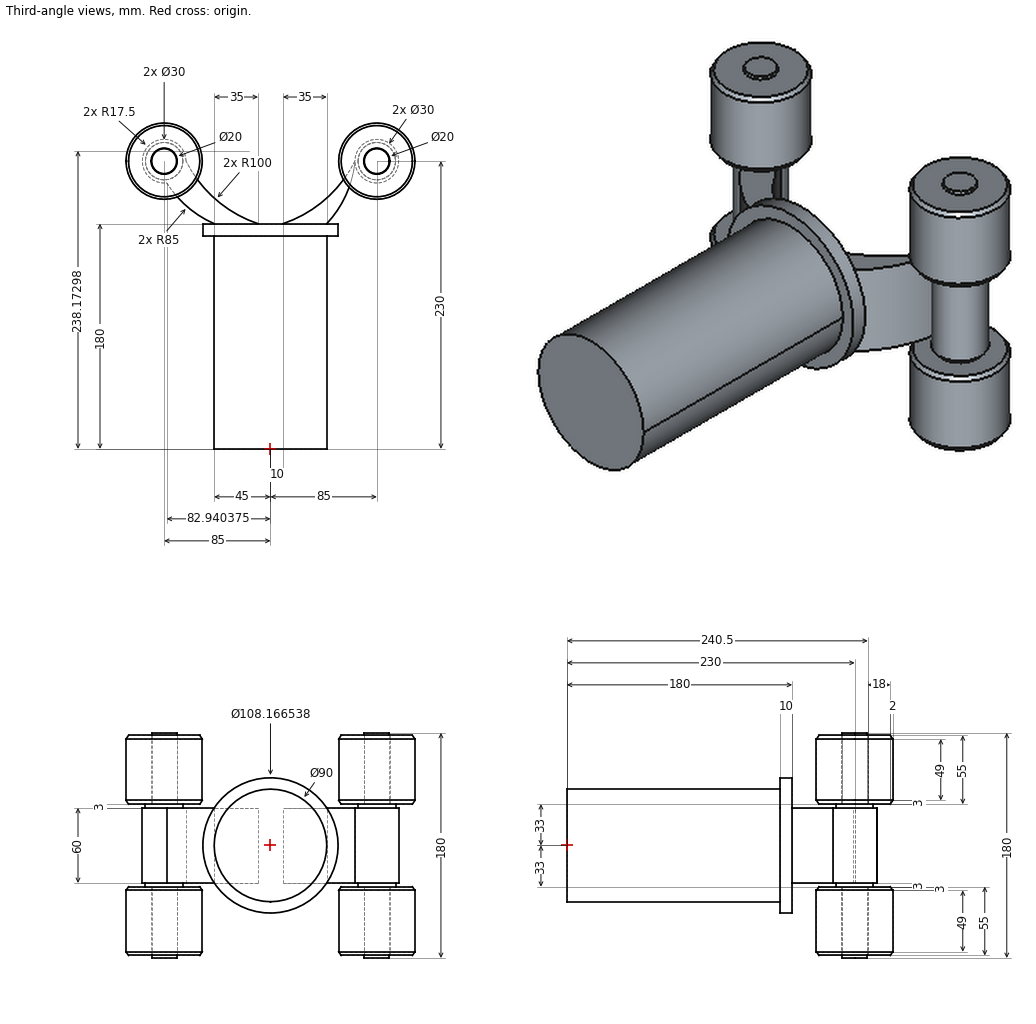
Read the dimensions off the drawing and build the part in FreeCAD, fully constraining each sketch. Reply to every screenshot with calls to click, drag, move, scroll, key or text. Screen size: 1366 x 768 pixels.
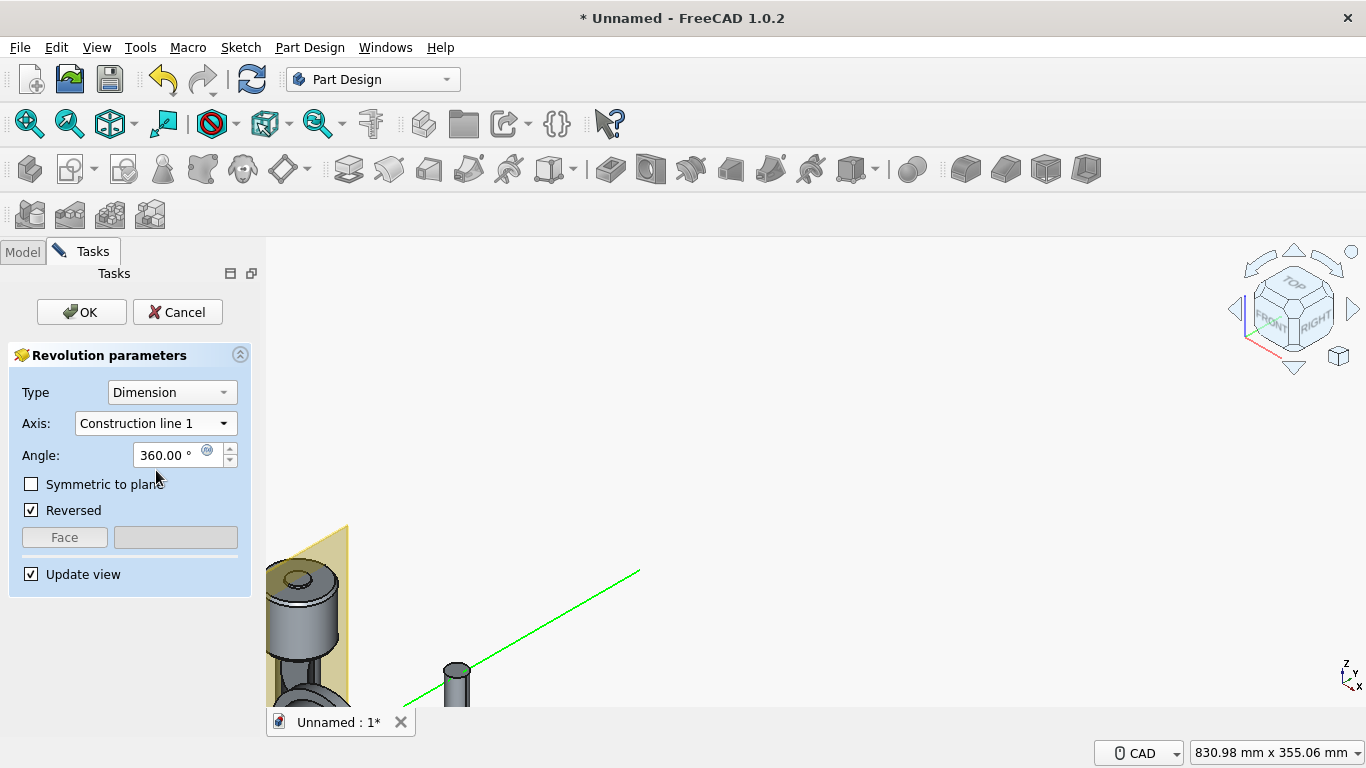
click(82, 312)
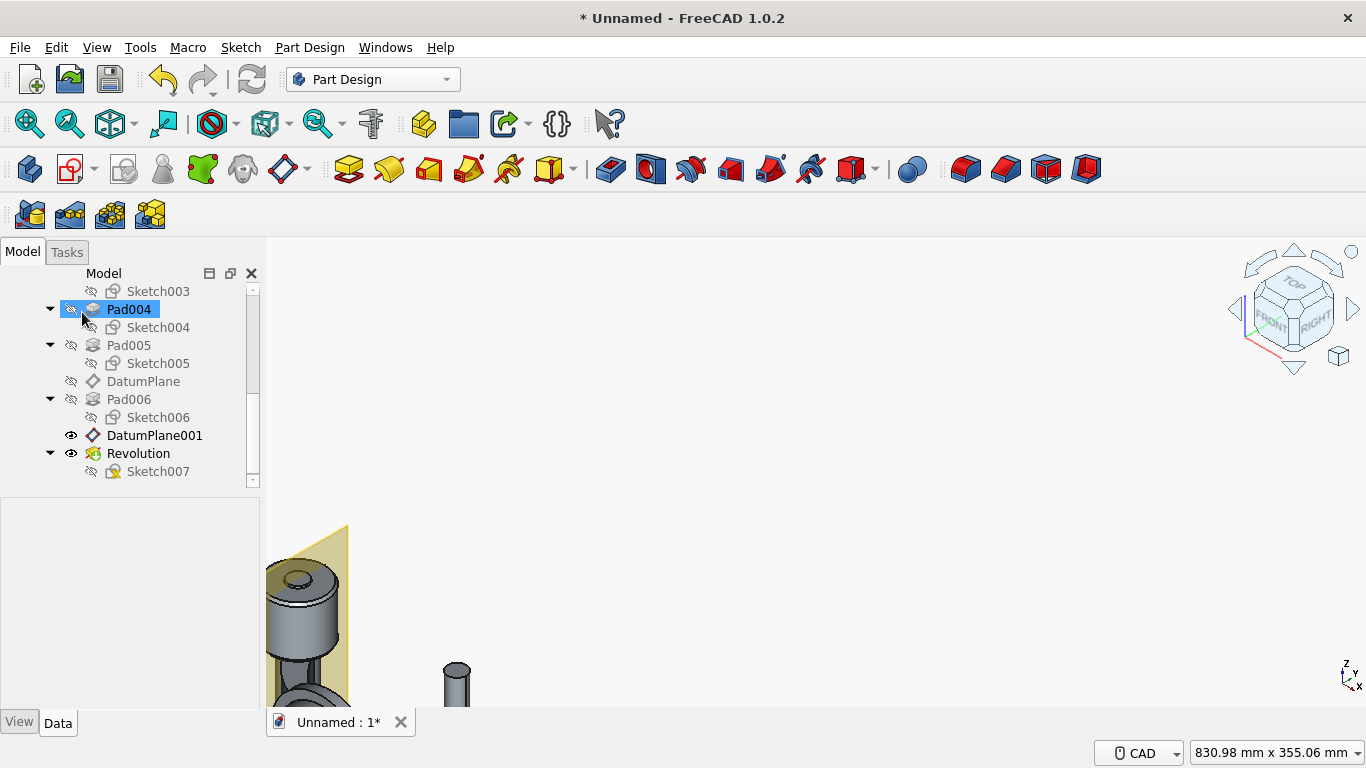
click(116, 435)
key(space)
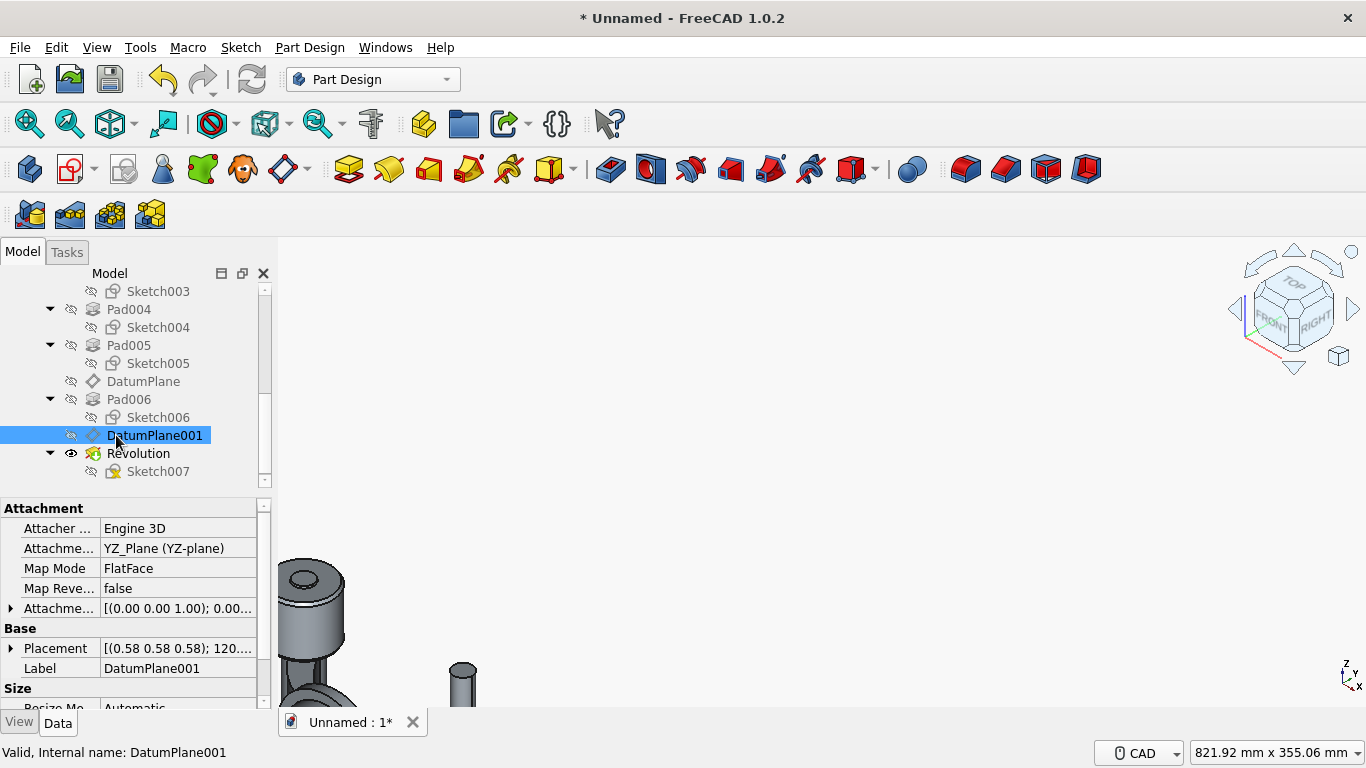
click(30, 124)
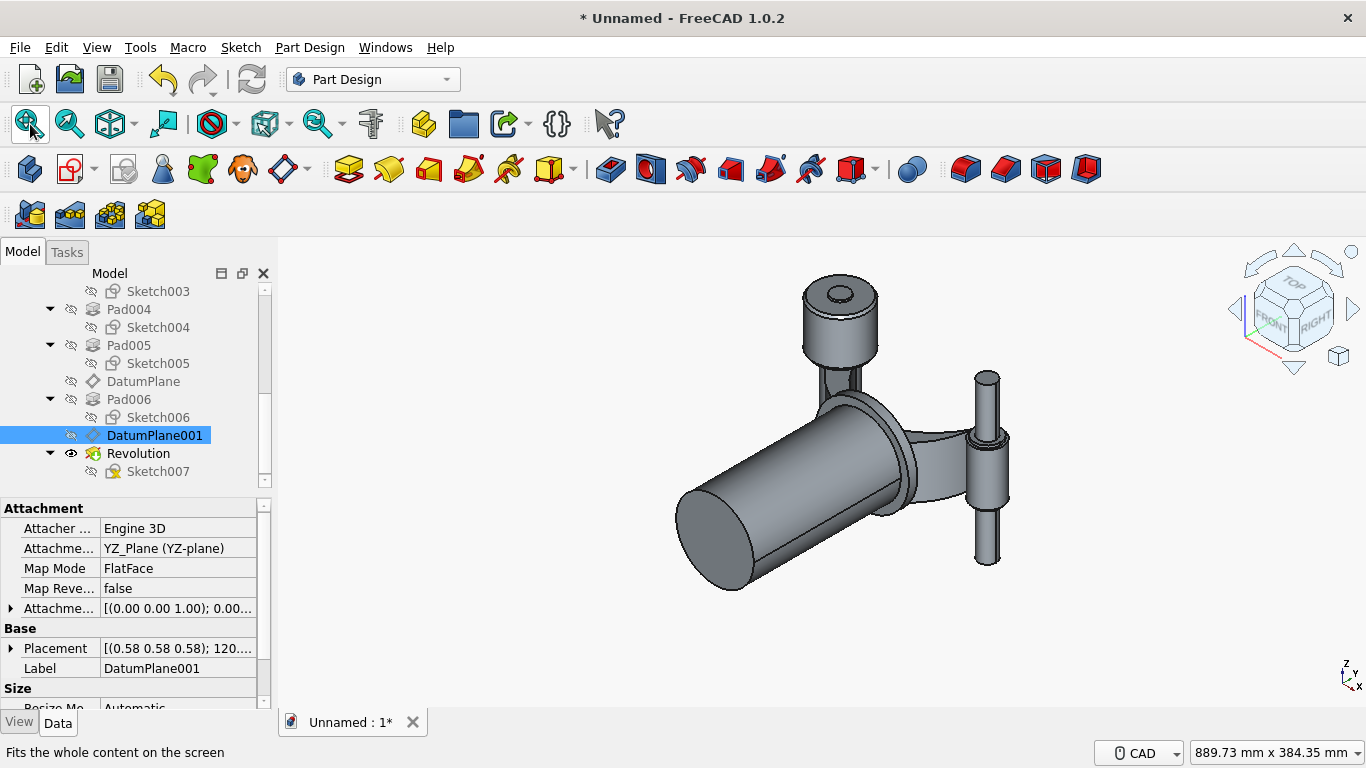
click(116, 453)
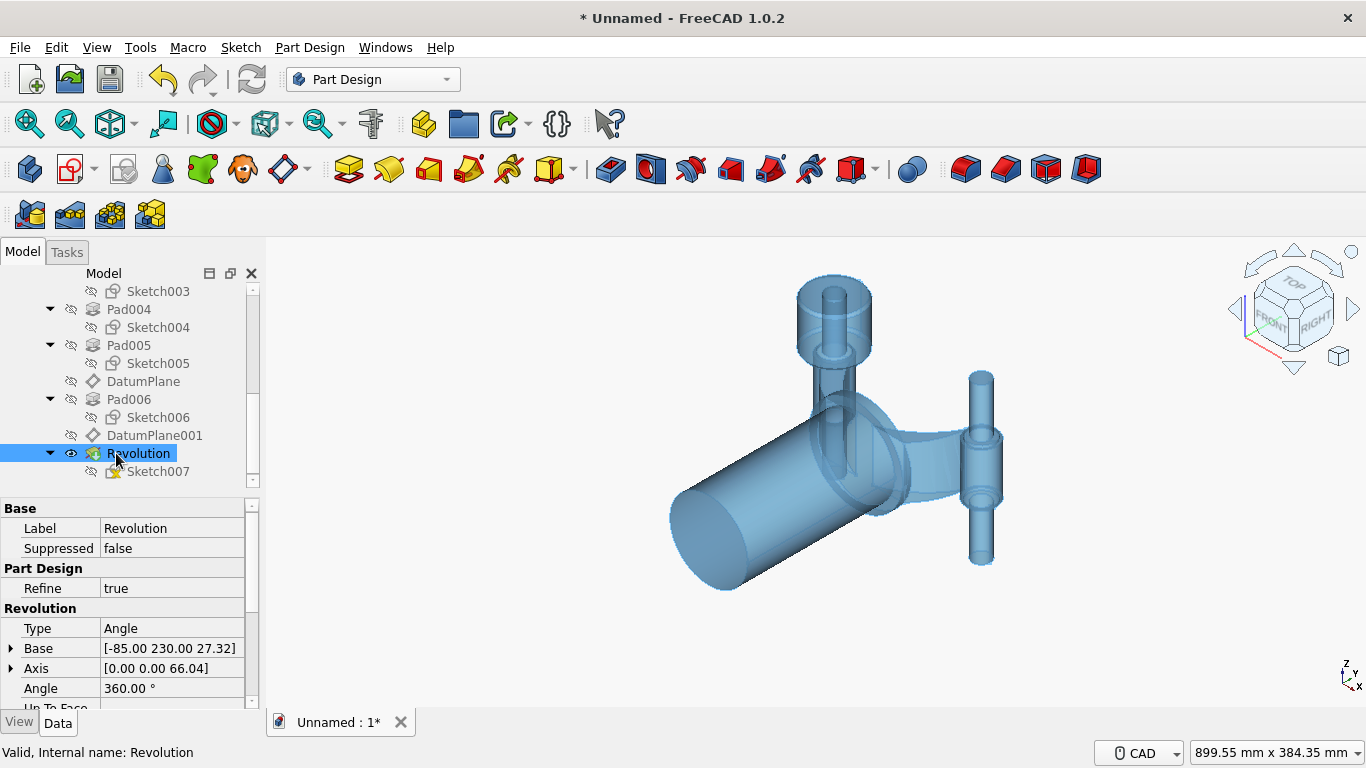
click(30, 214)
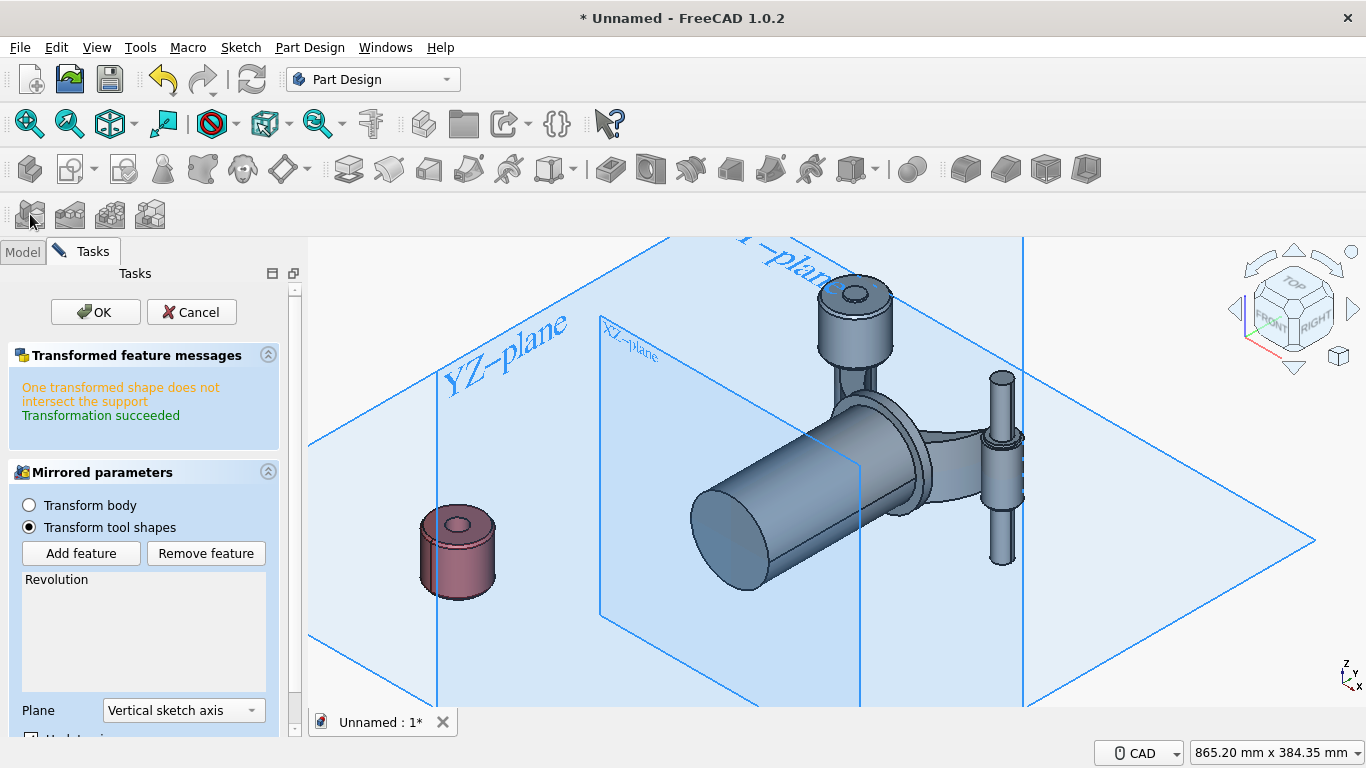
click(184, 710)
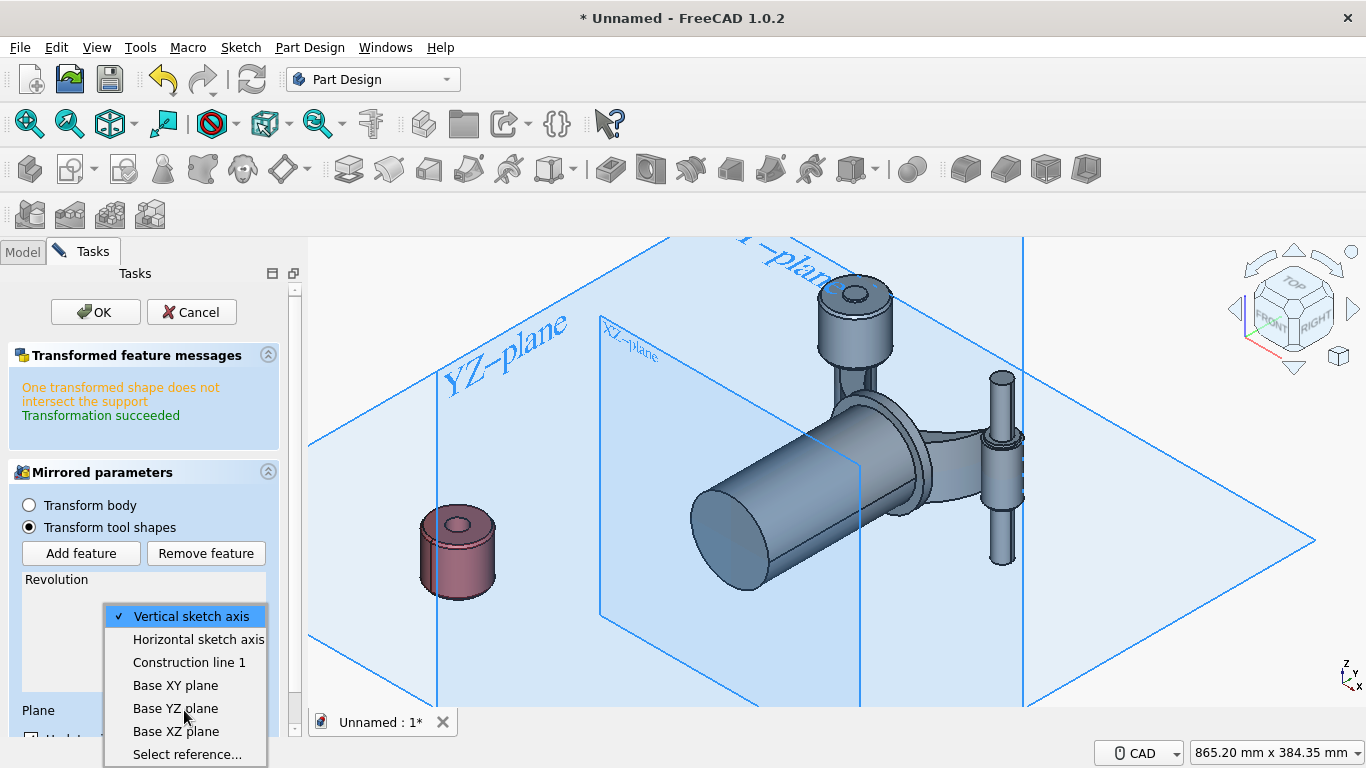
click(184, 708)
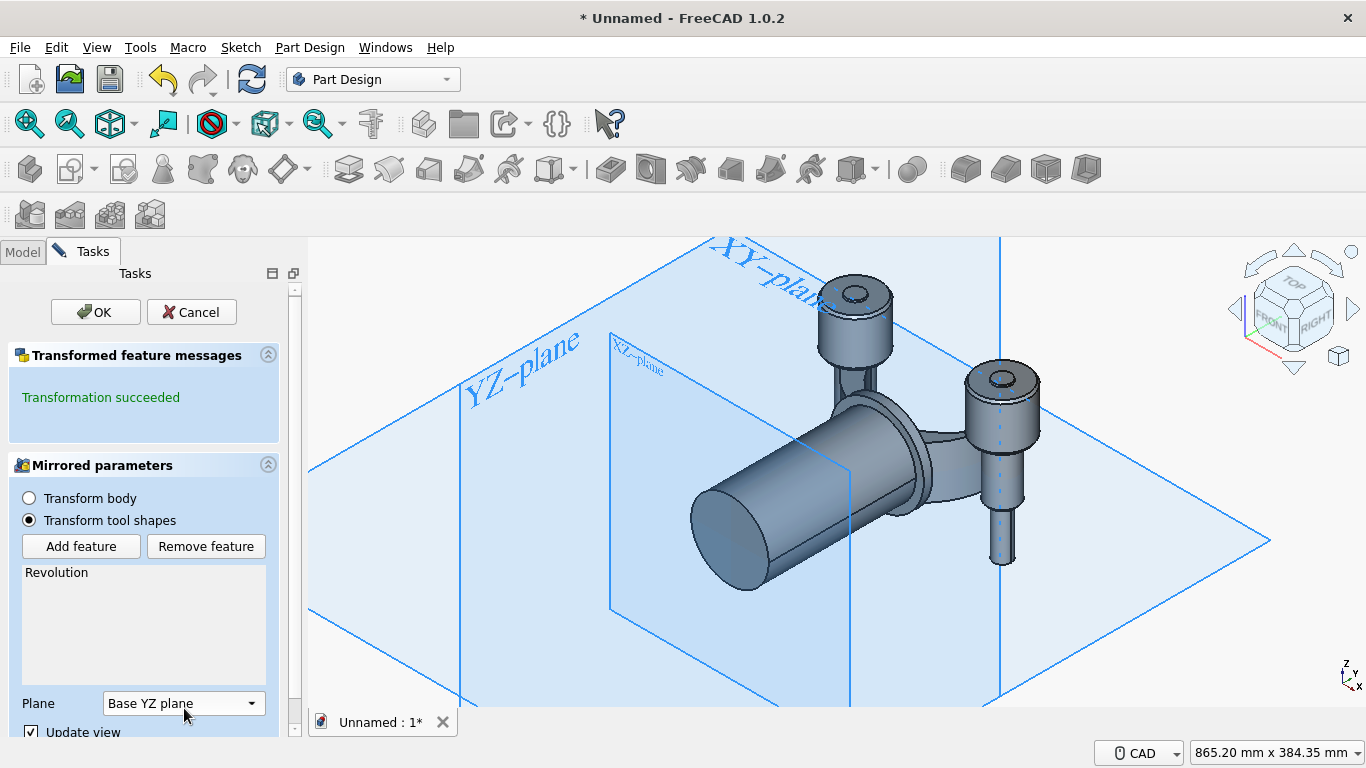
click(96, 312)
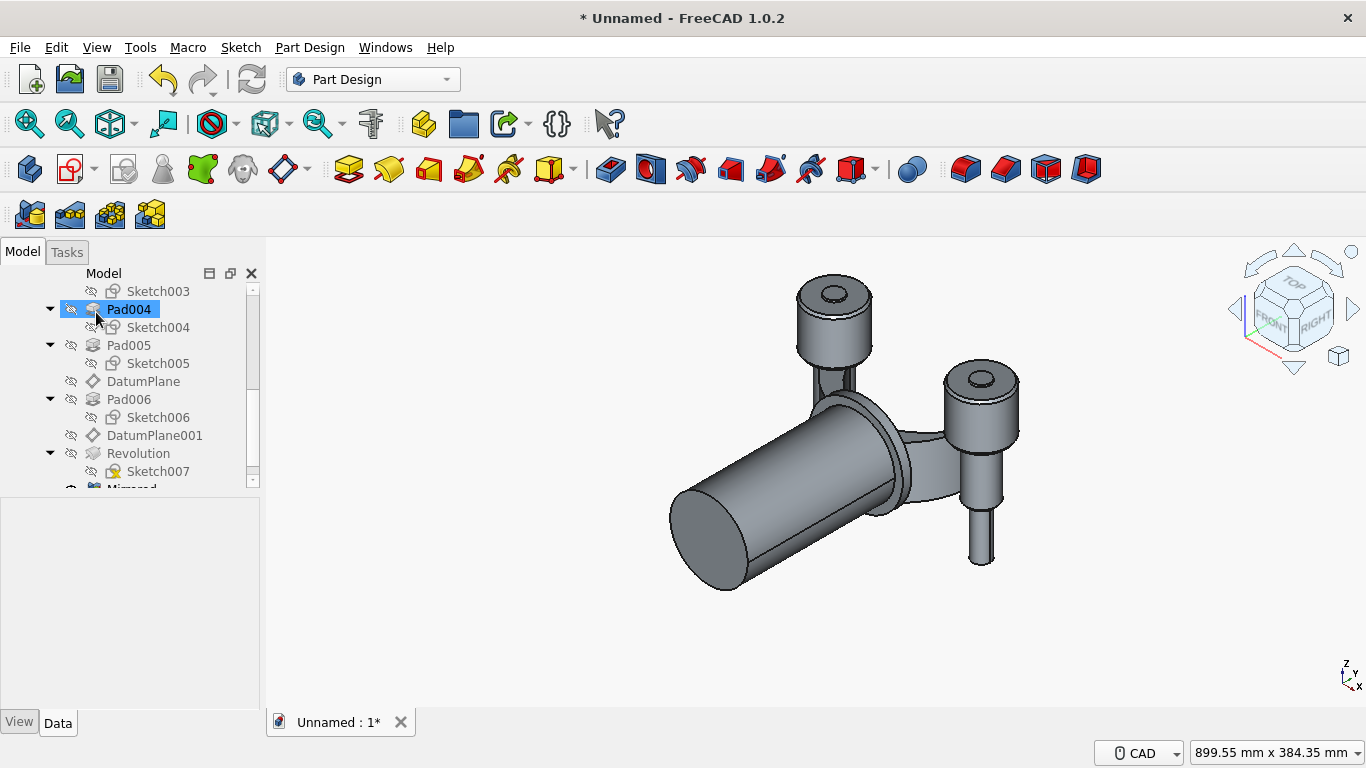
click(116, 453)